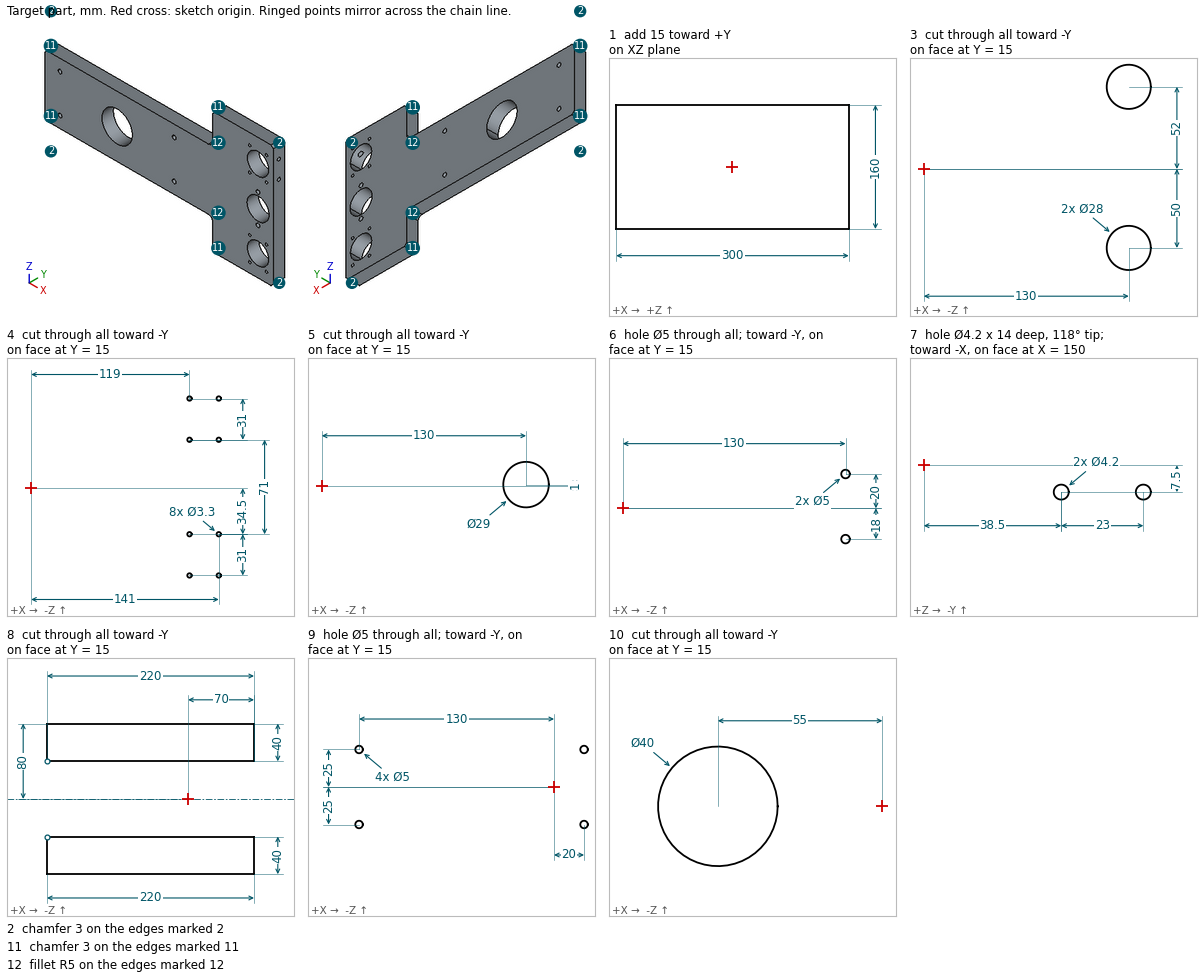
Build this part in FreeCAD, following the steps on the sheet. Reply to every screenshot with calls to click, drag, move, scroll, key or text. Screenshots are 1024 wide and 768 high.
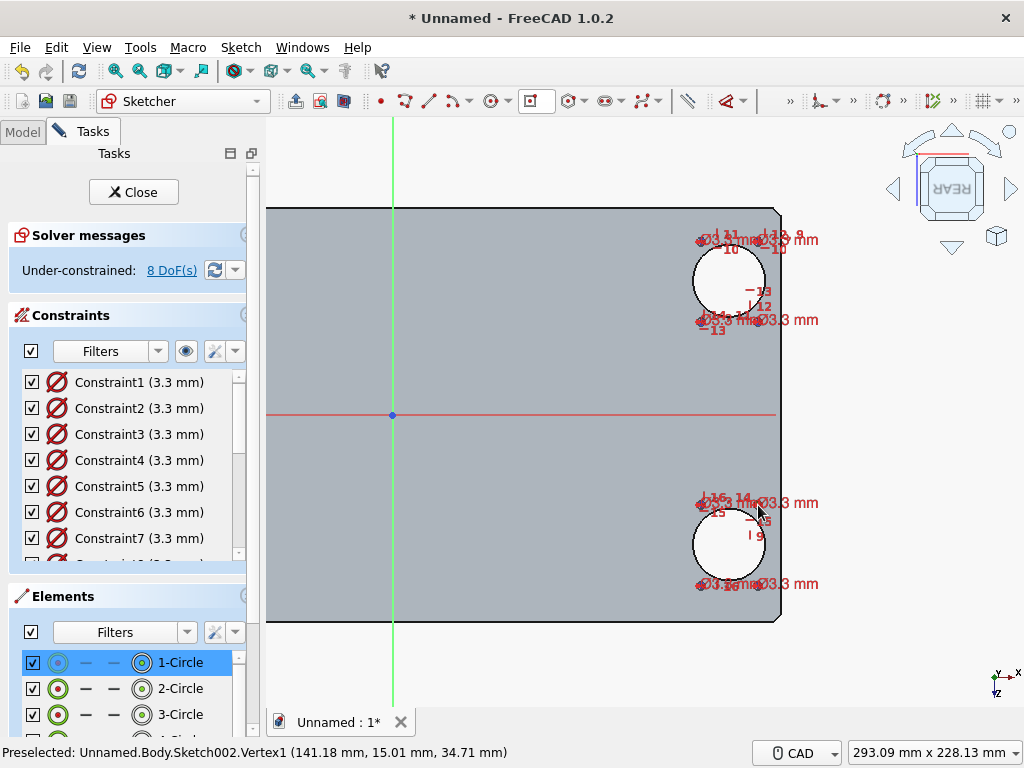
click(758, 586)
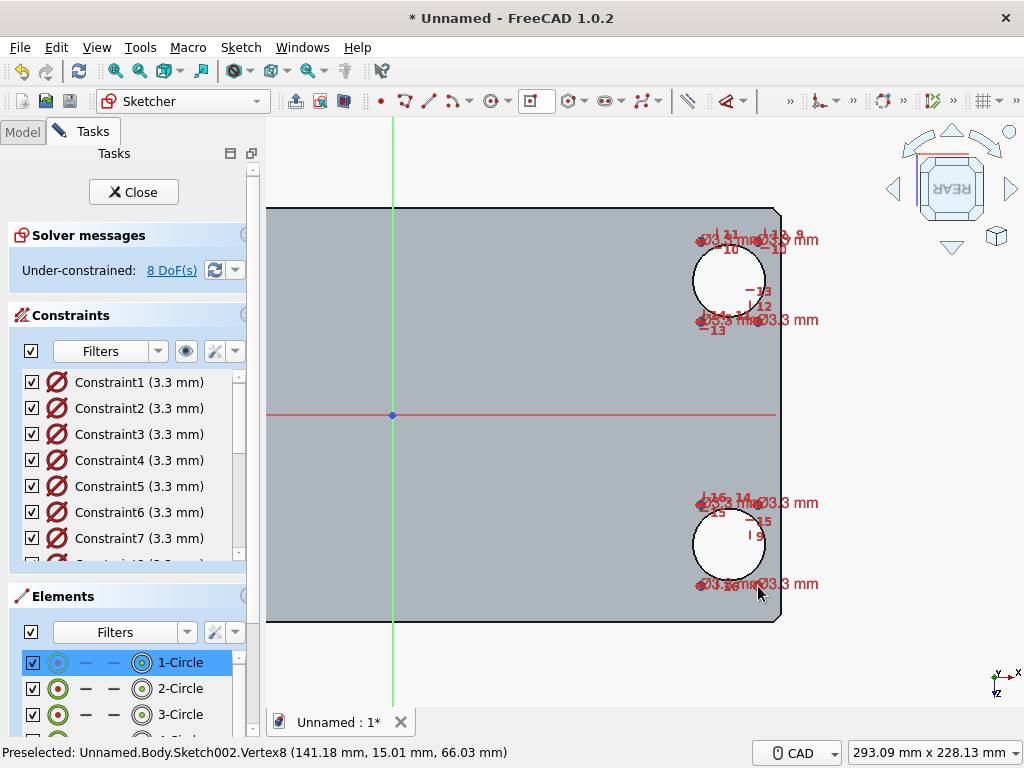
key(v)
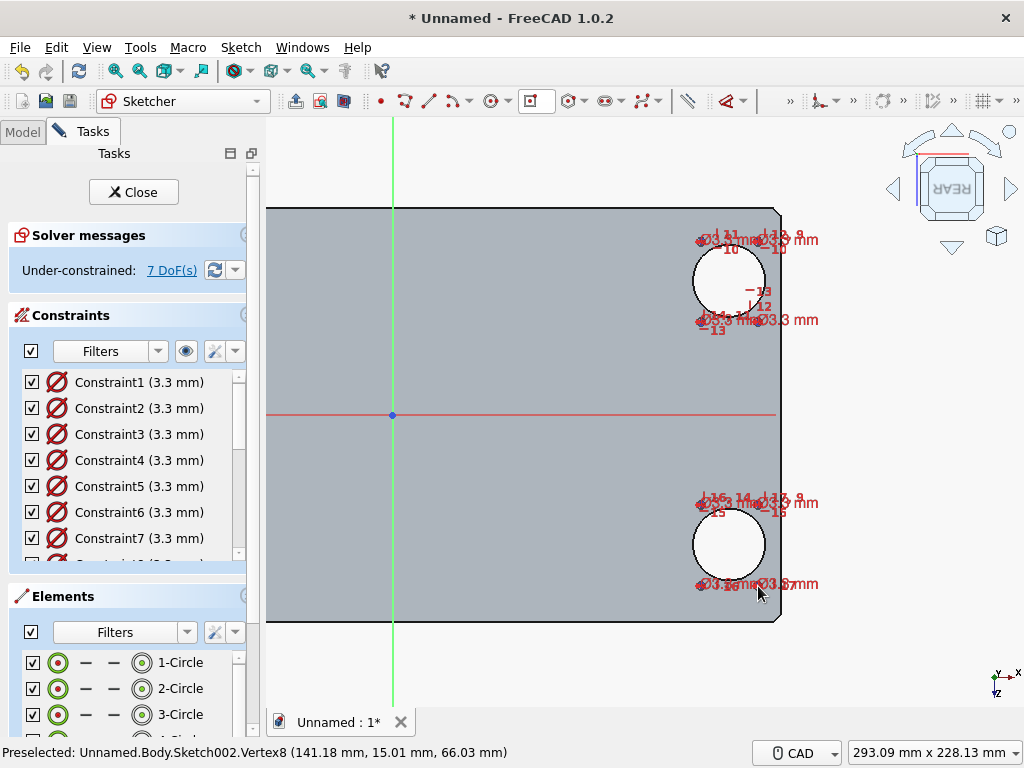
click(701, 586)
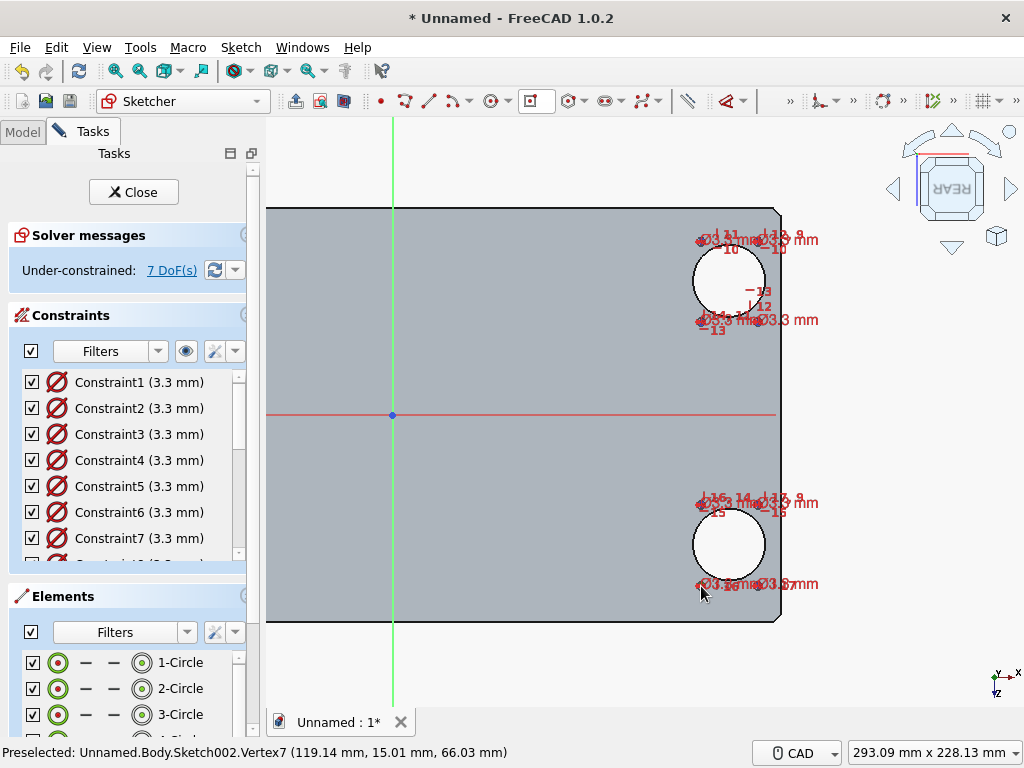
click(758, 586)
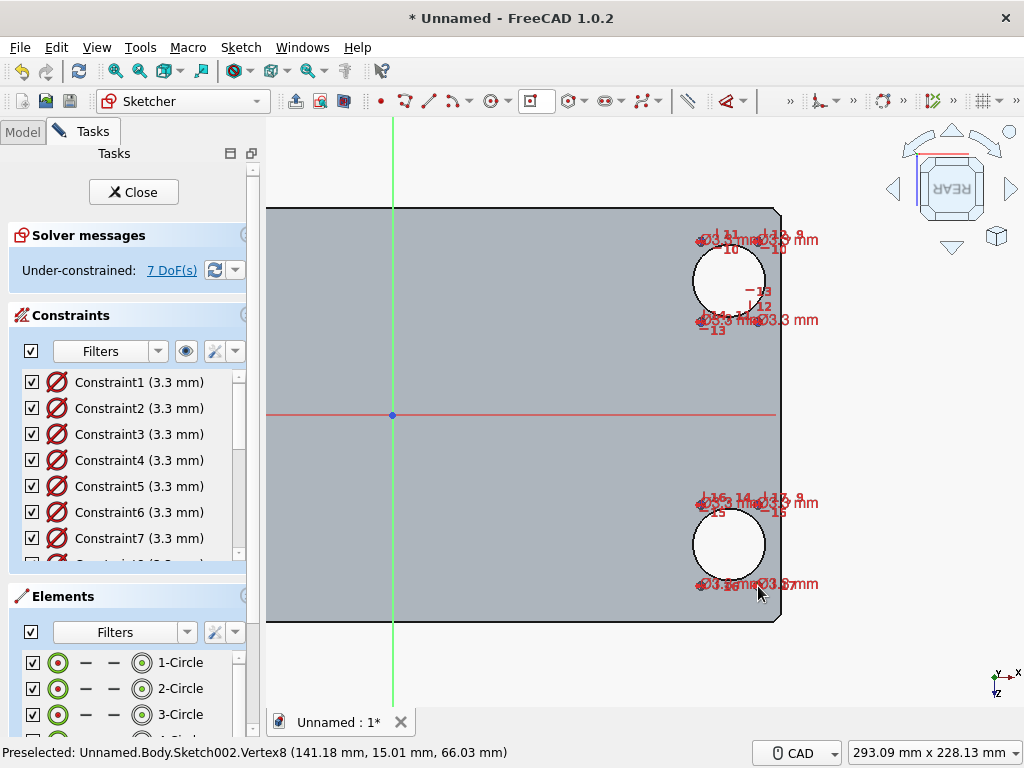
key(h)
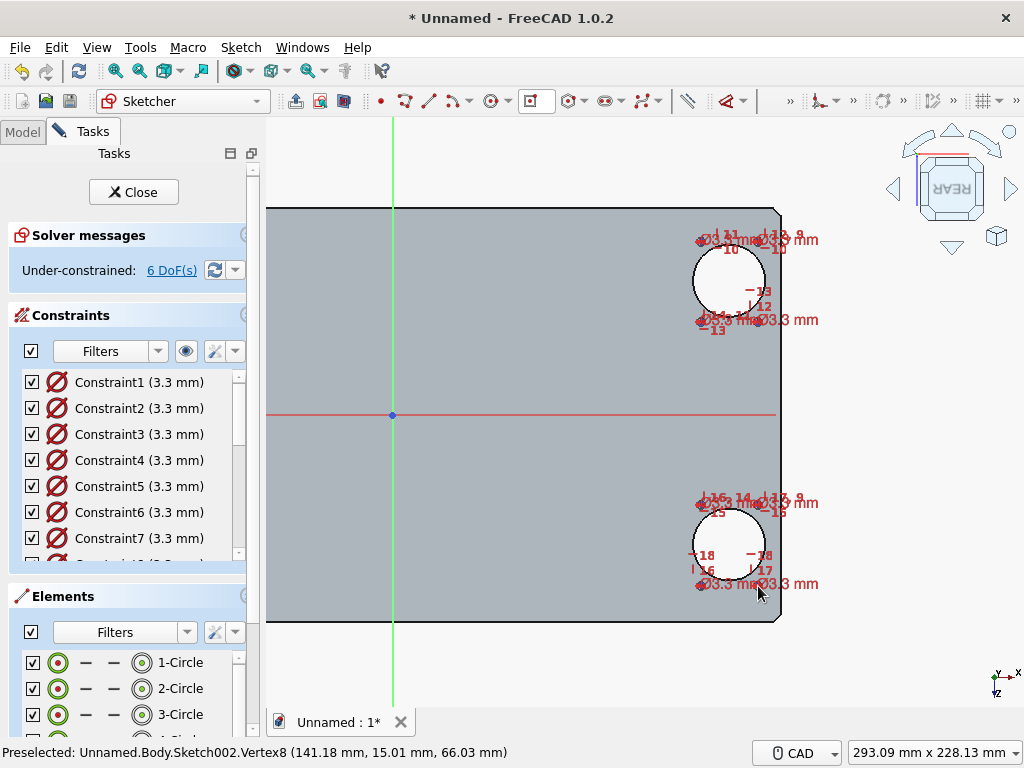
click(726, 102)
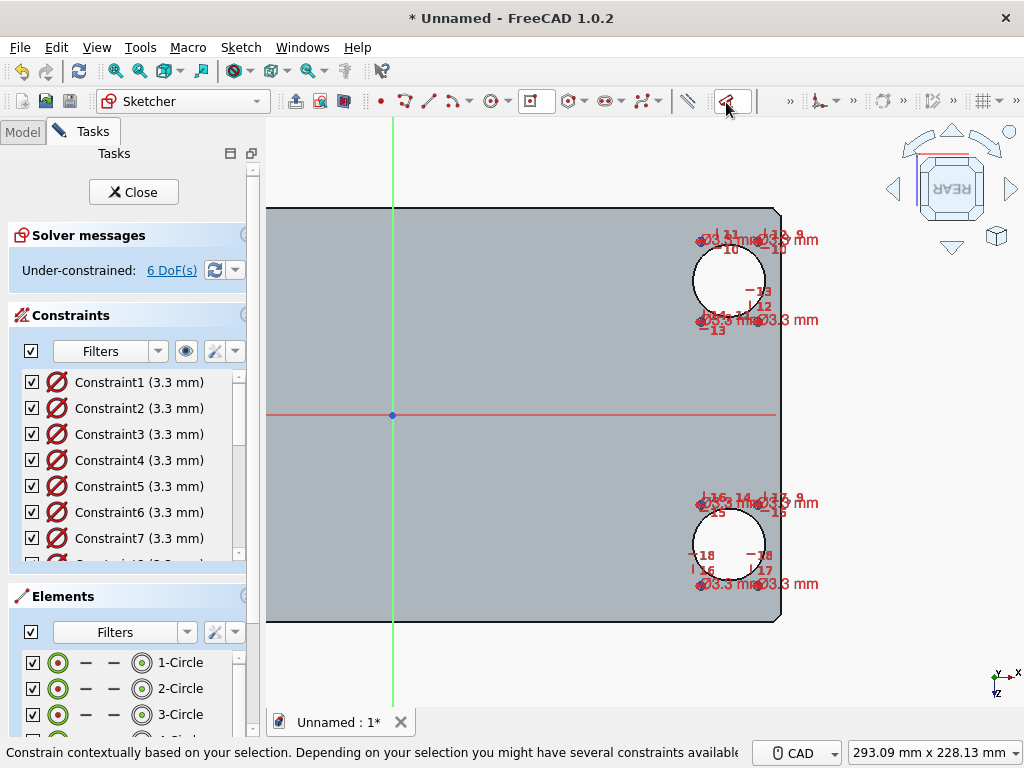
click(758, 505)
click(575, 539)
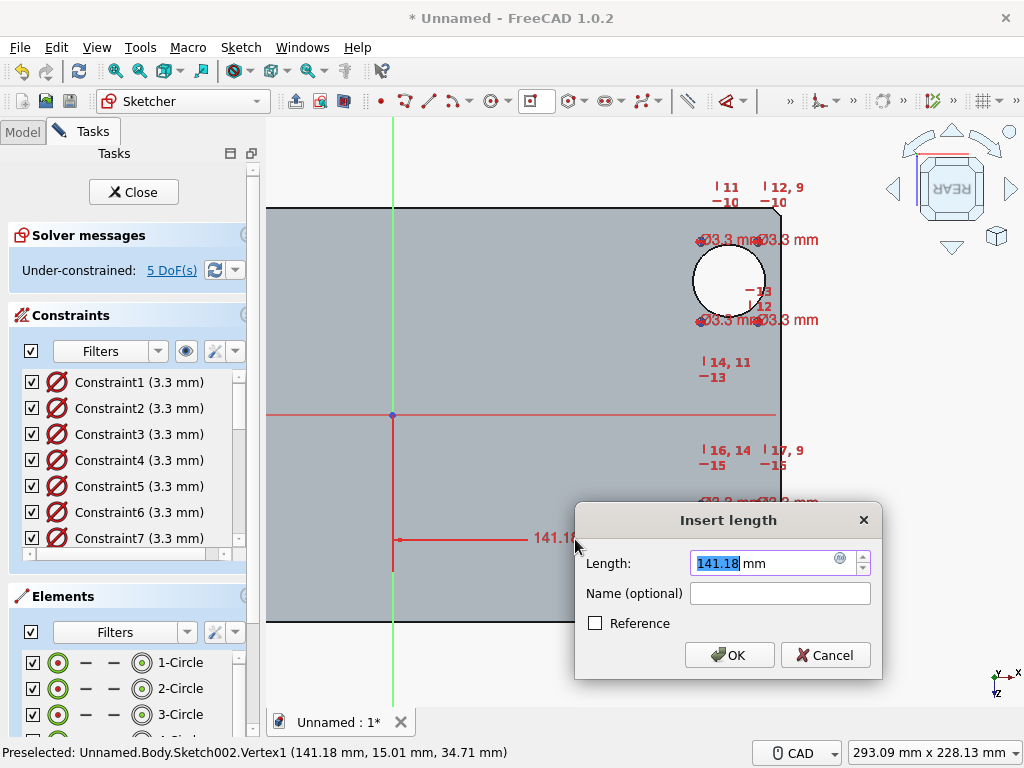
text(141)
key(Return)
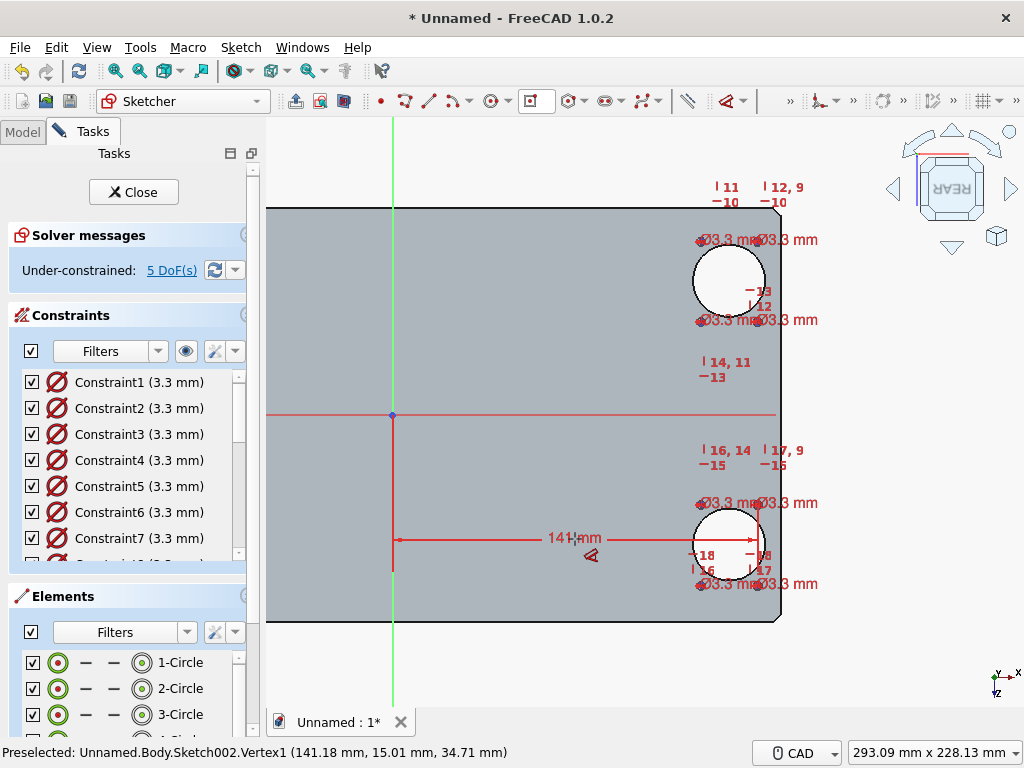
click(701, 242)
click(547, 208)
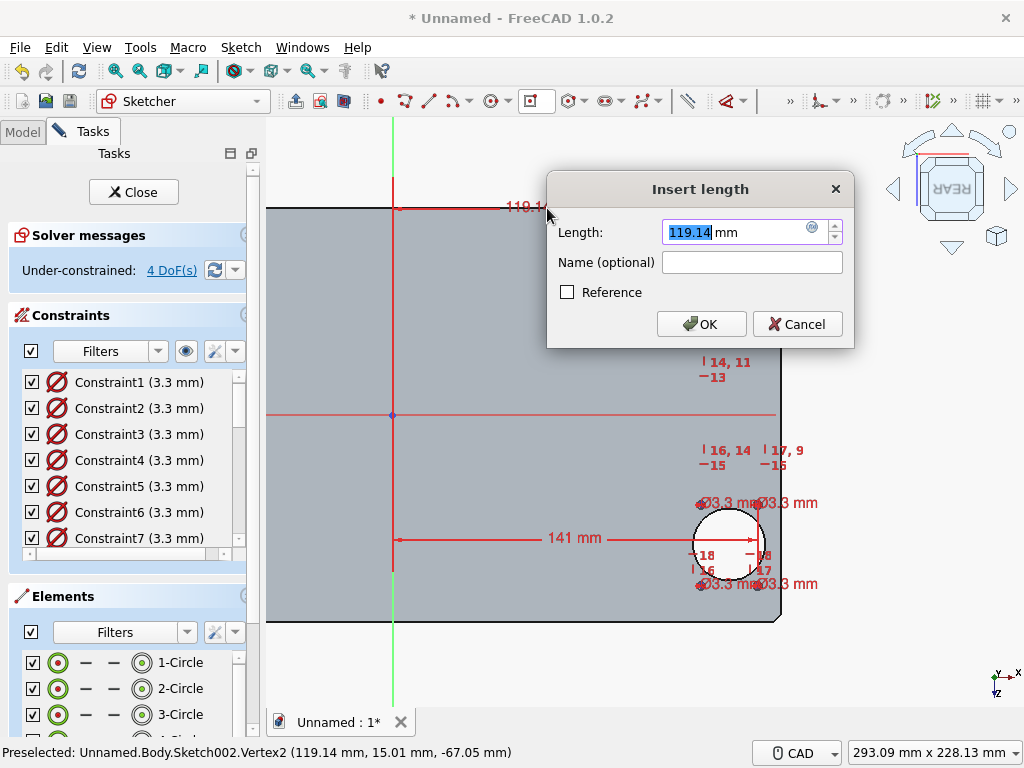
text(119)
key(Return)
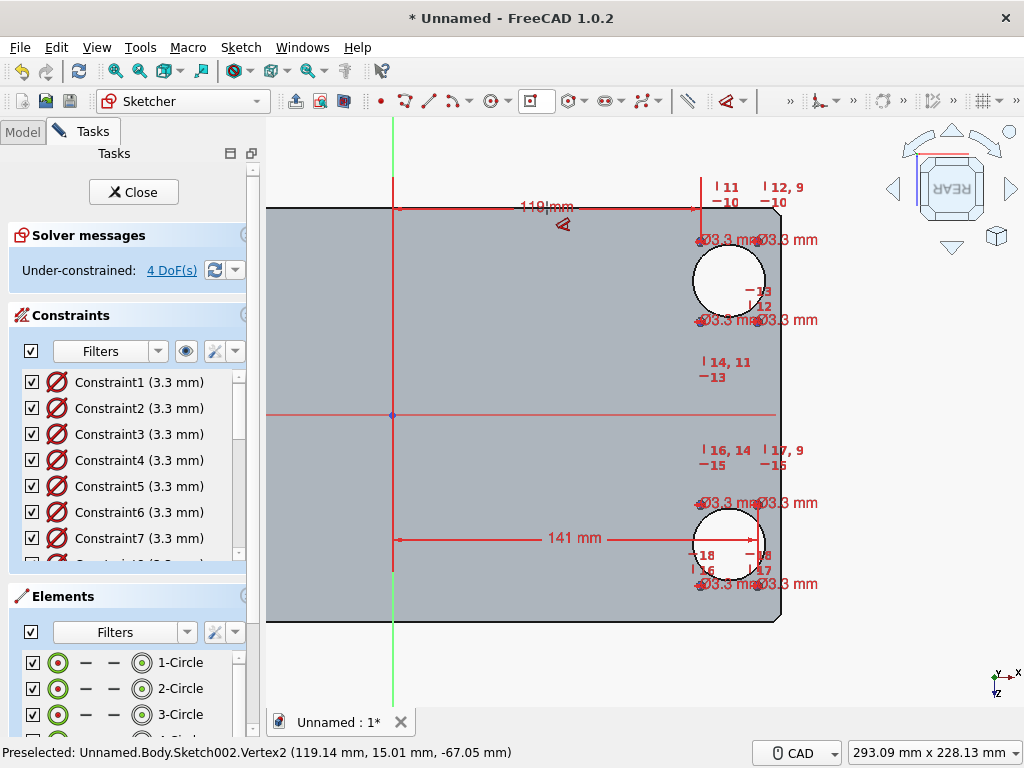
click(701, 242)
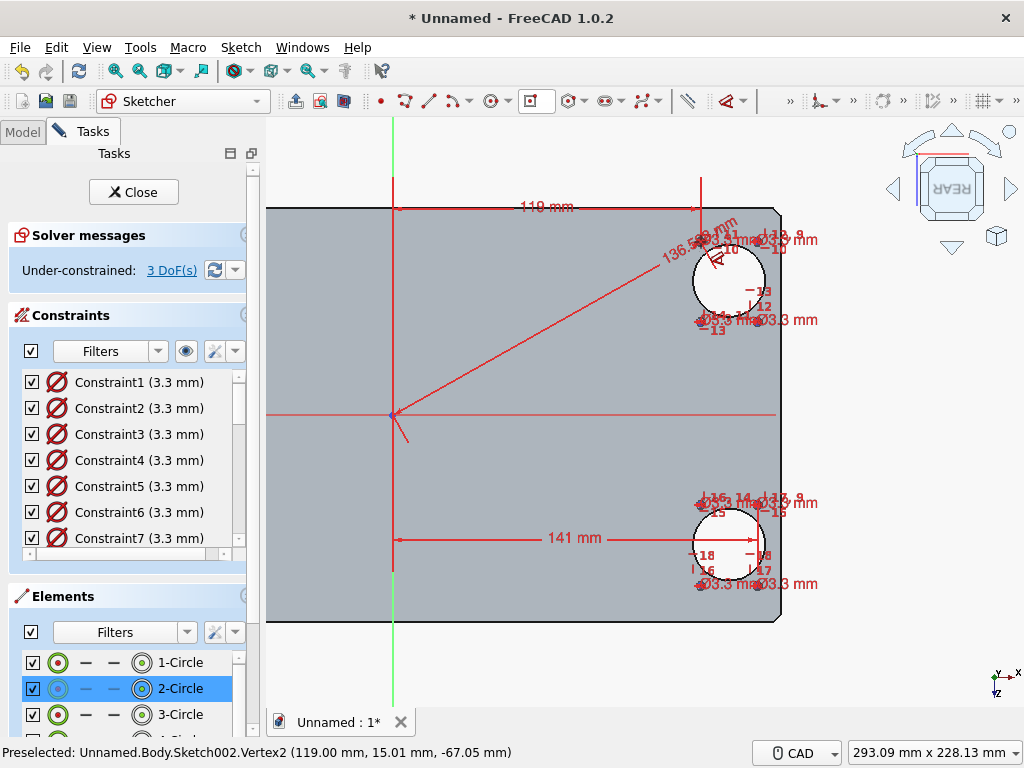
click(701, 322)
click(735, 282)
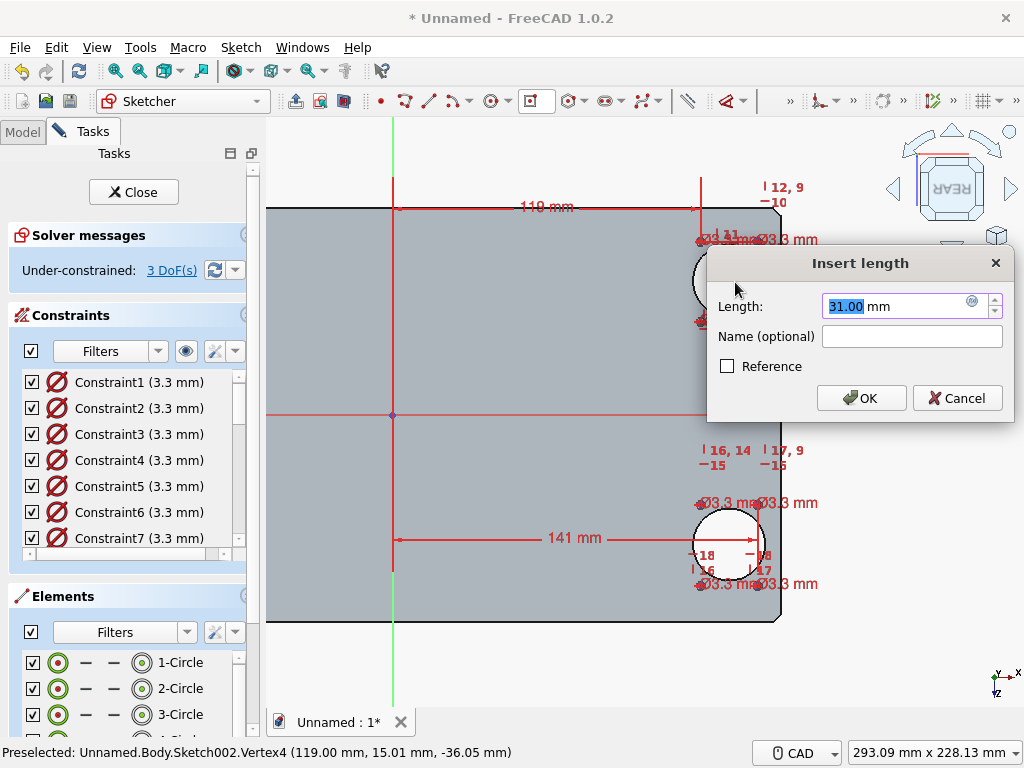
text(31)
key(Return)